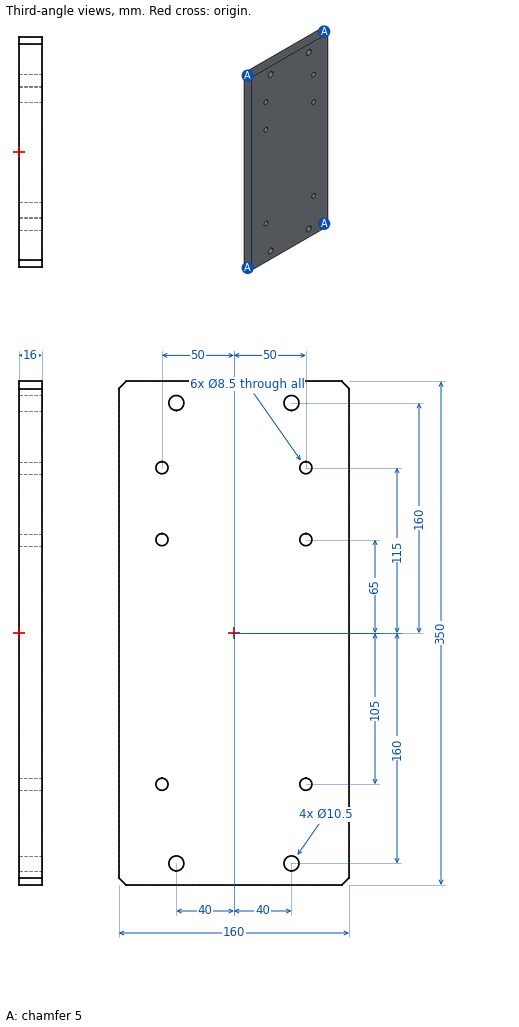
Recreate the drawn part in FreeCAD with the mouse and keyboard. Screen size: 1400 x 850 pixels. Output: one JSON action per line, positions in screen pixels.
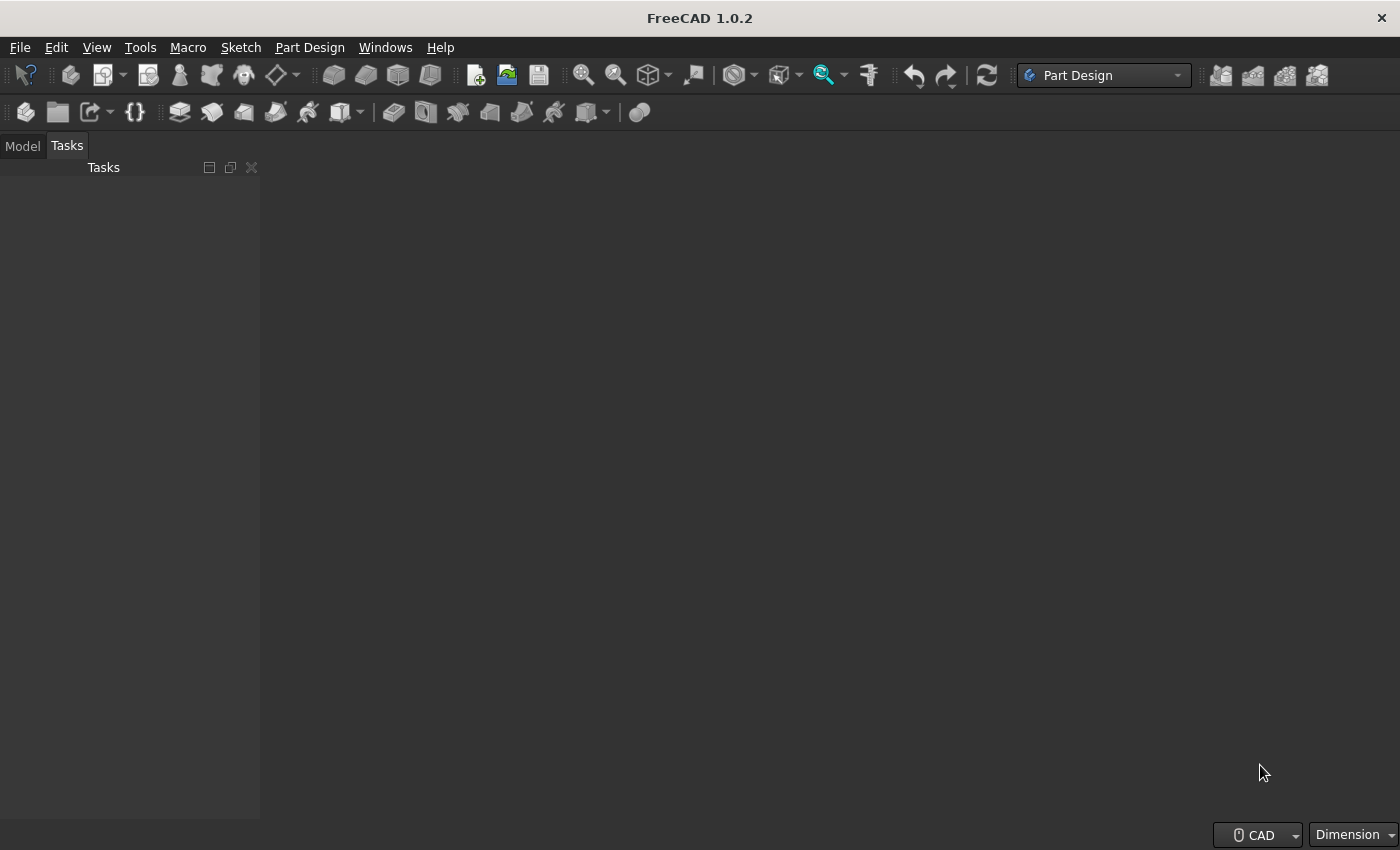
{"action": "key", "text": "ctrl+n"}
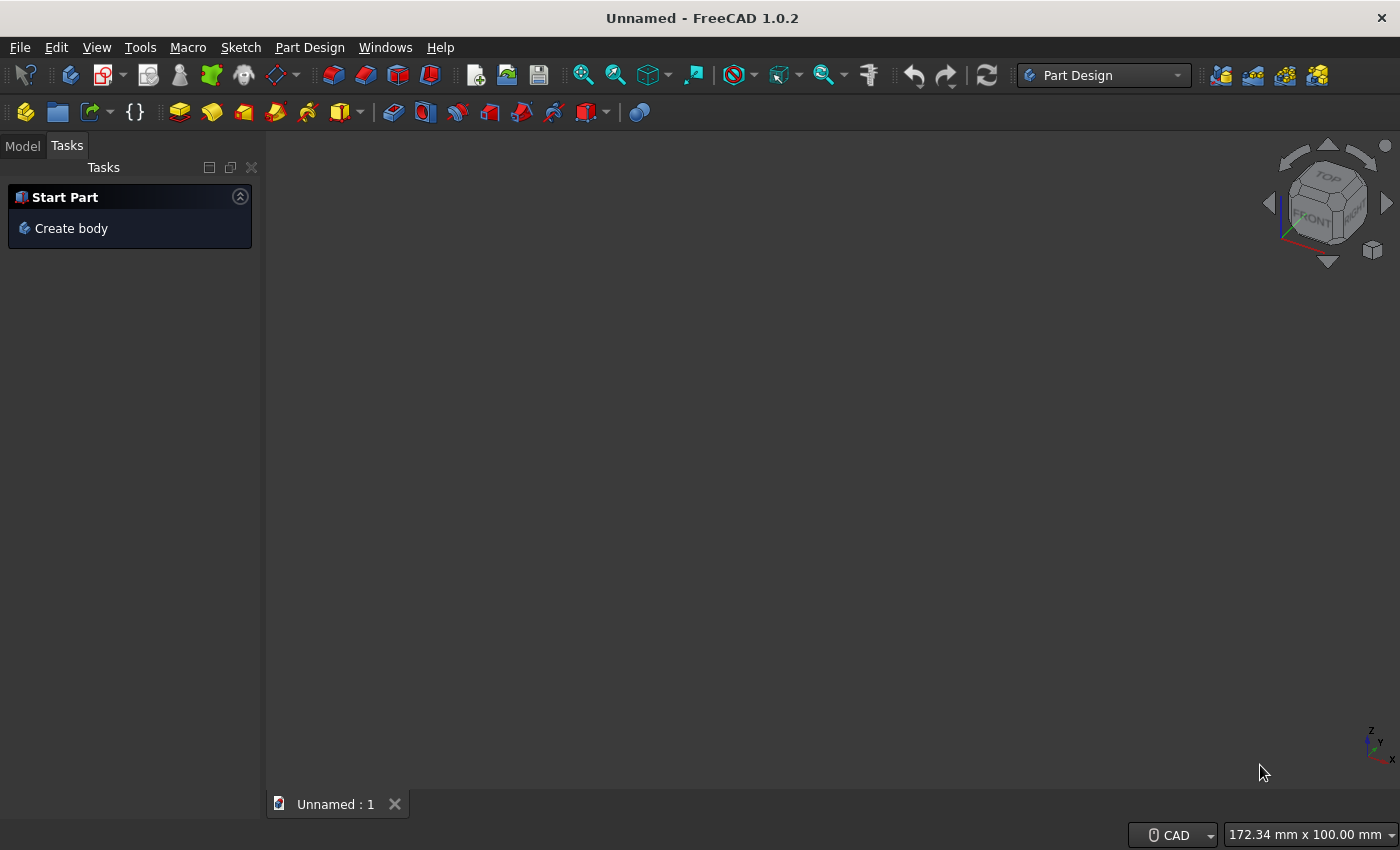
{"action": "left_click", "coordinate": [104, 76]}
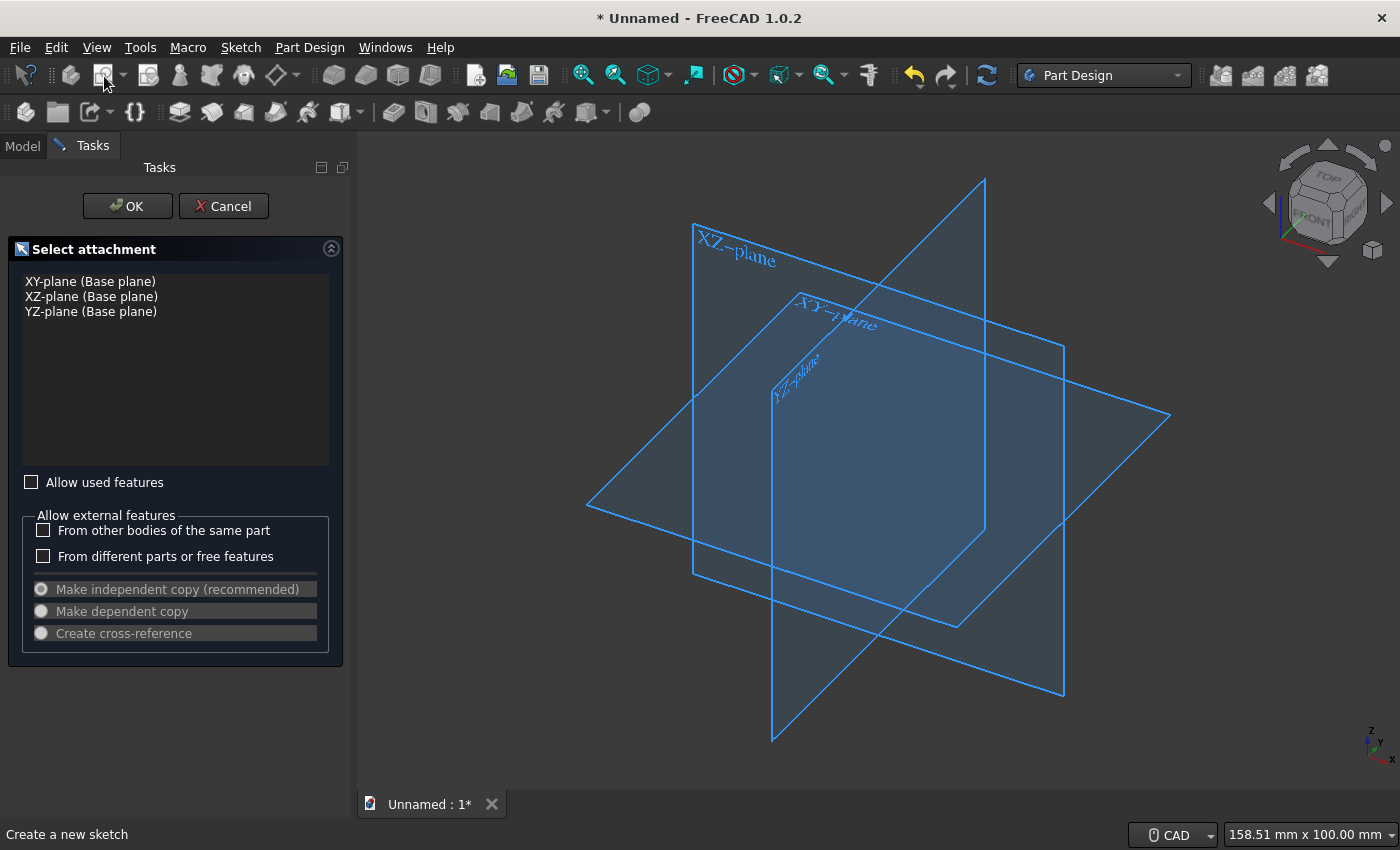
{"action": "left_click", "coordinate": [82, 312]}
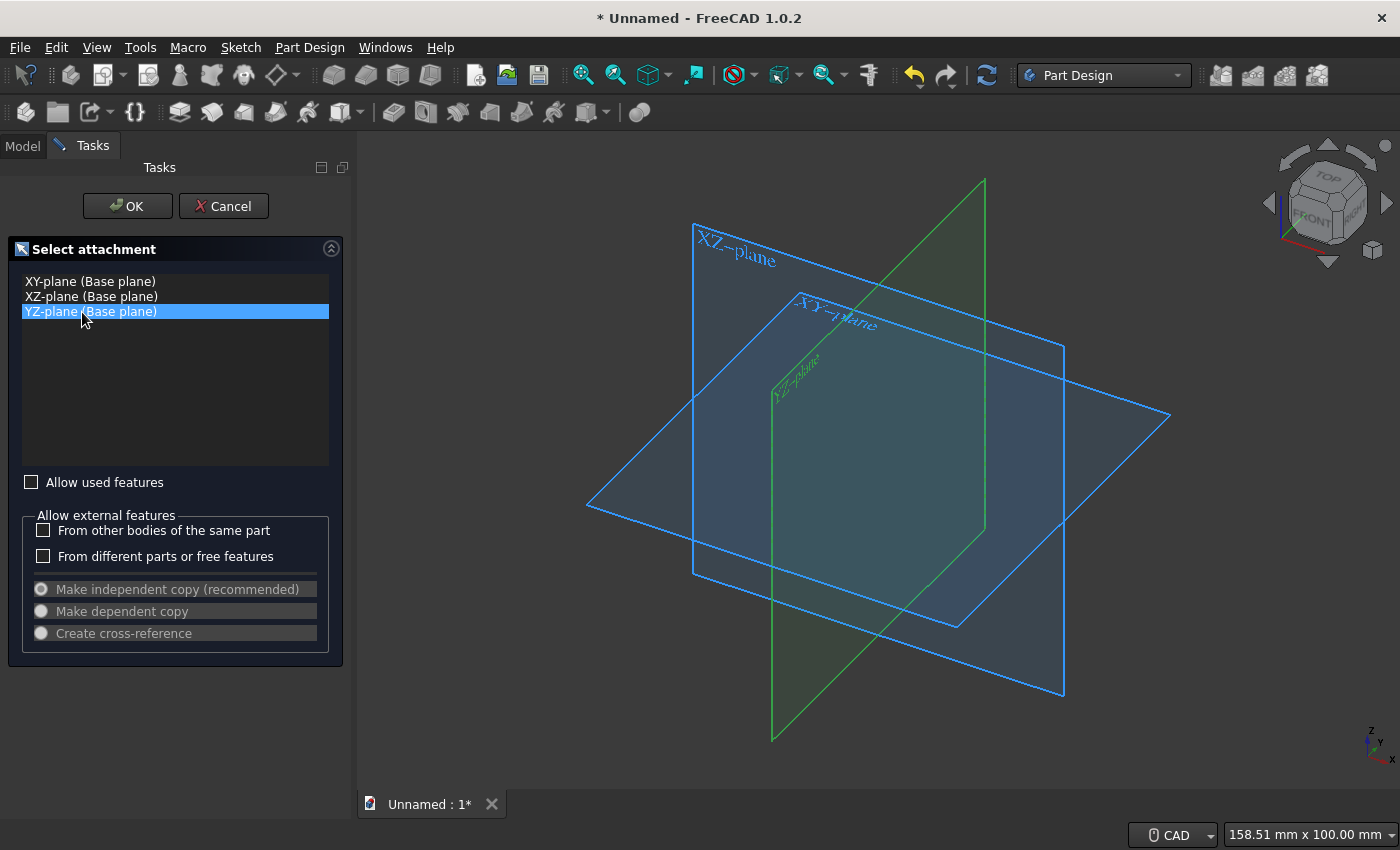
{"action": "left_click", "coordinate": [128, 206]}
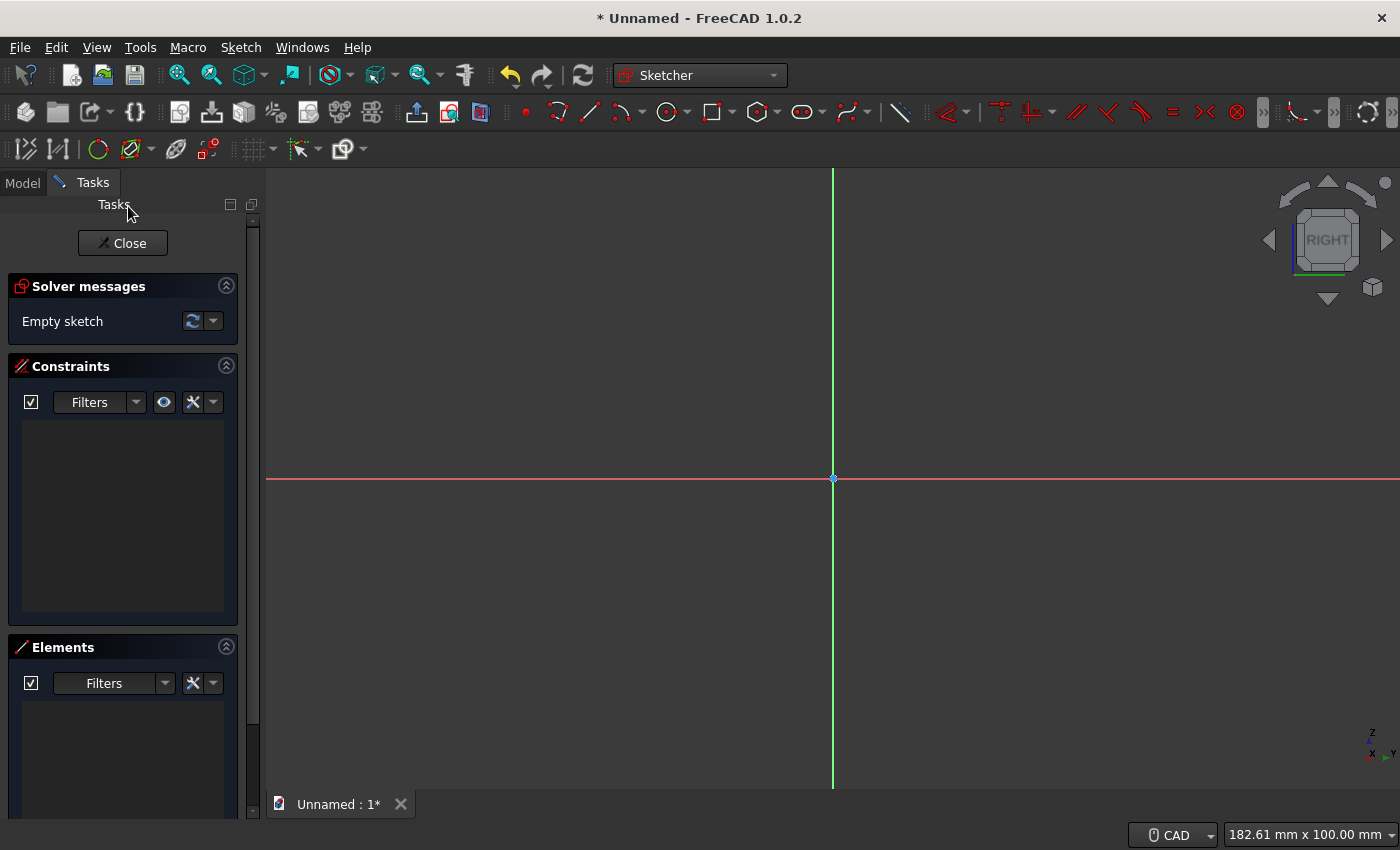
{"action": "scroll", "coordinate": [747, 478], "scroll_direction": "down", "scroll_amount": 8}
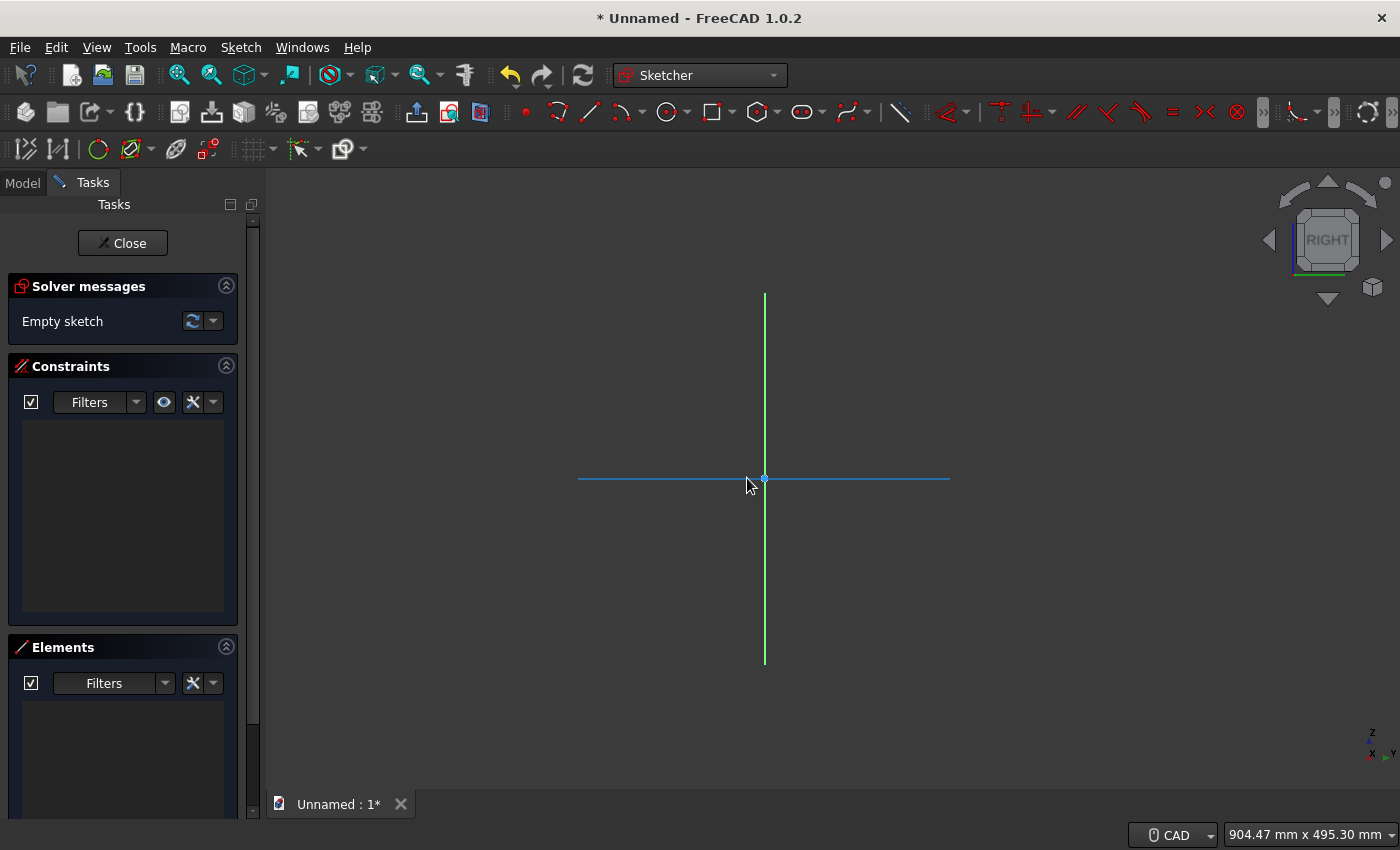
{"action": "key", "text": "g v"}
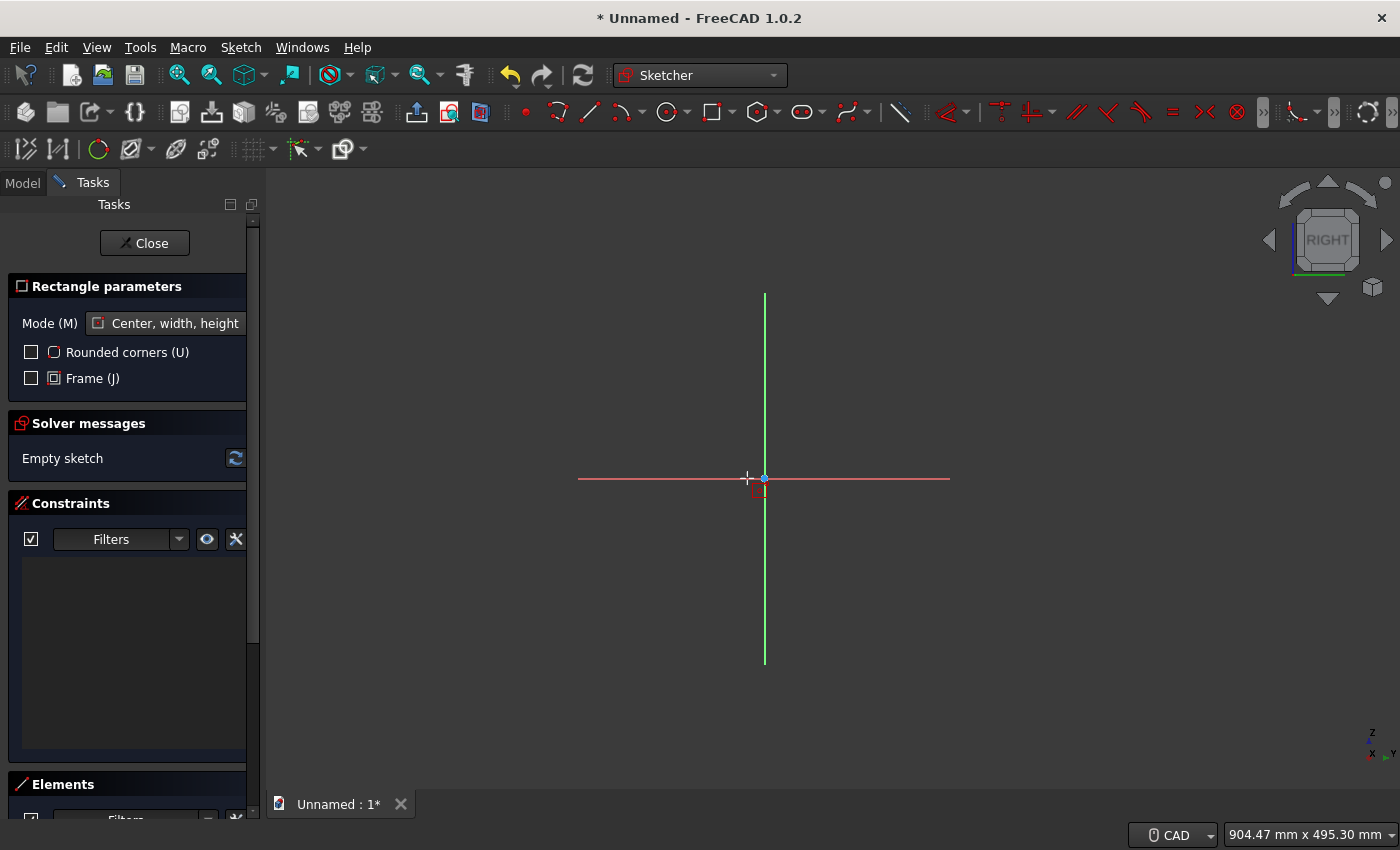
{"action": "left_click", "coordinate": [765, 478]}
{"action": "mouse_move", "coordinate": [865, 259]}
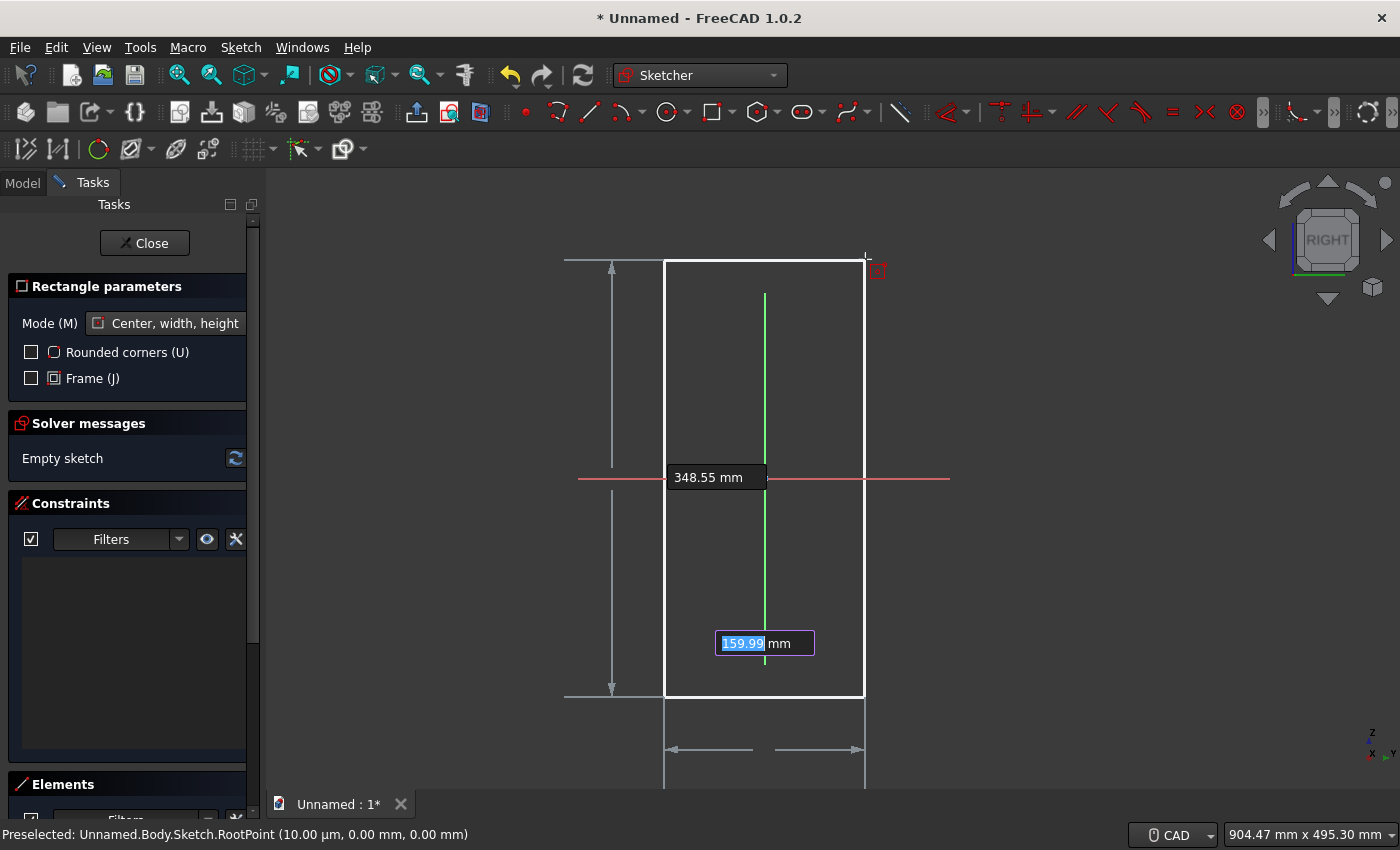
{"action": "type", "text": "160"}
{"action": "key", "text": "Tab"}
{"action": "type", "text": "350"}
{"action": "key", "text": "Return"}
{"action": "key", "text": "Escape"}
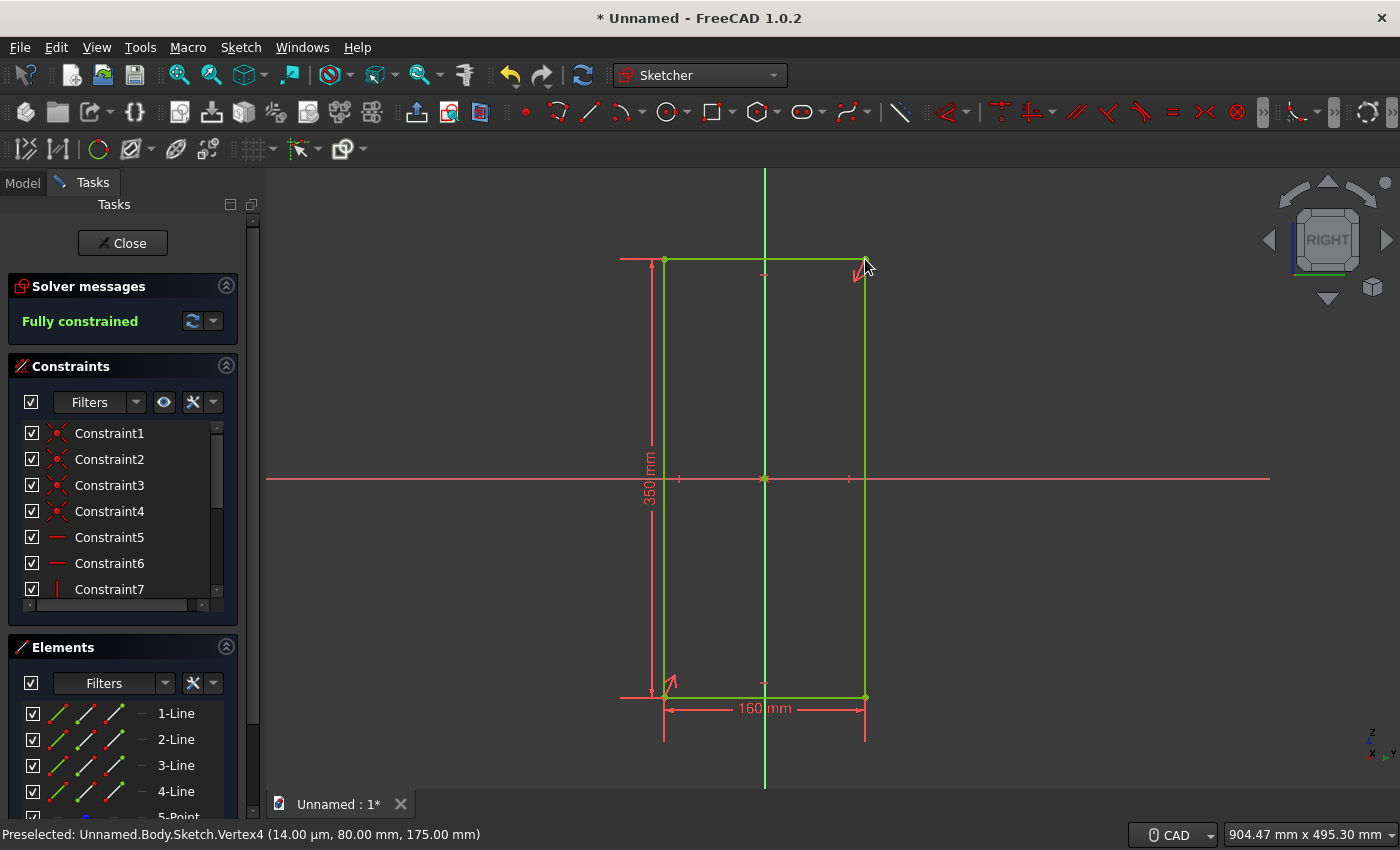
{"action": "left_click", "coordinate": [123, 243]}